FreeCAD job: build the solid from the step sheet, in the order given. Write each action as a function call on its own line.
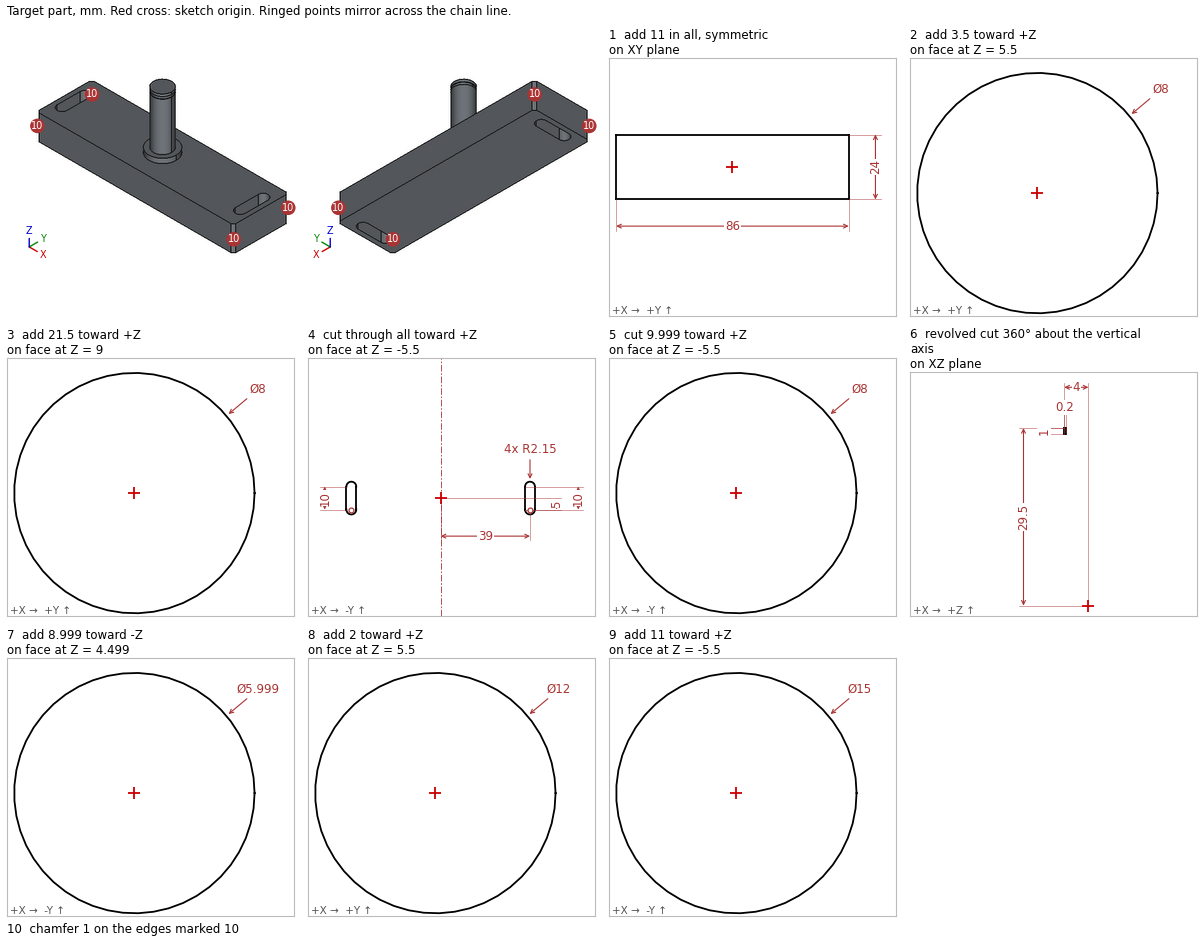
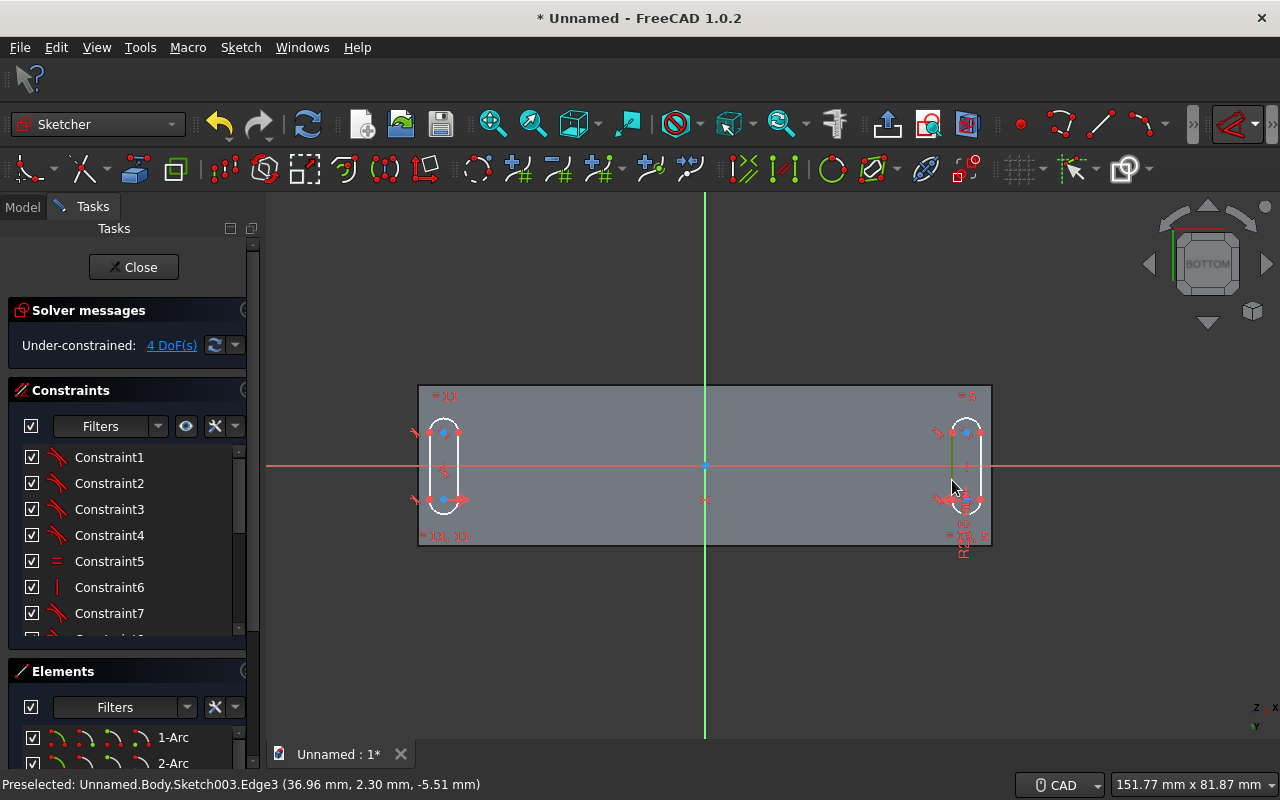
click(1258, 124)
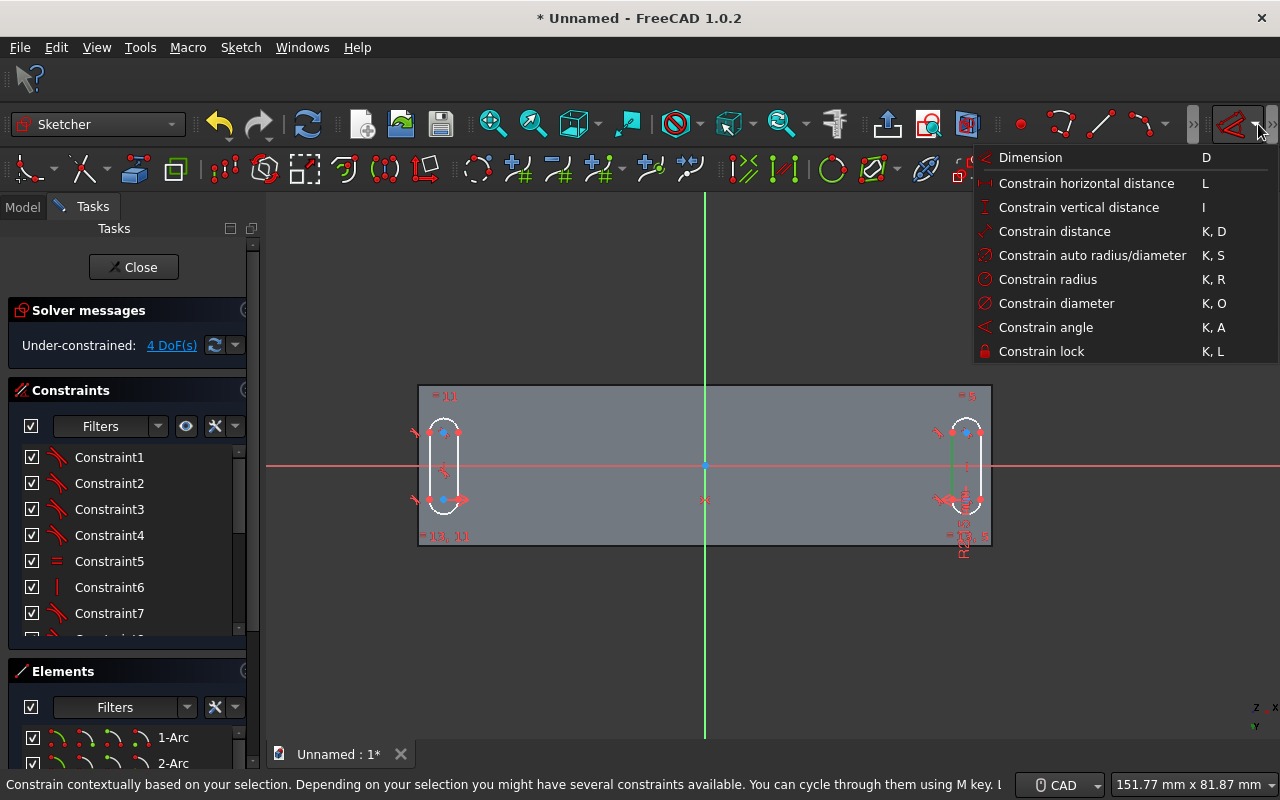
click(1126, 207)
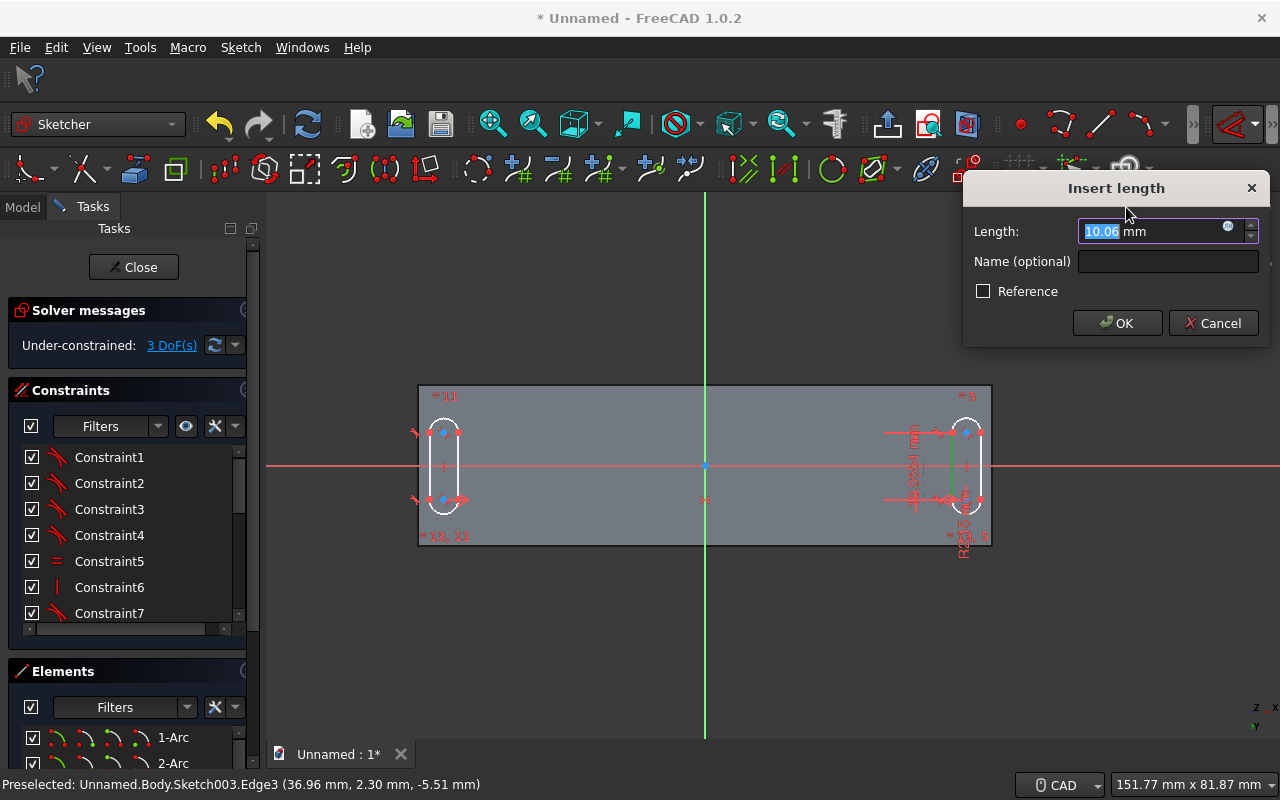
text(10)
key(Return)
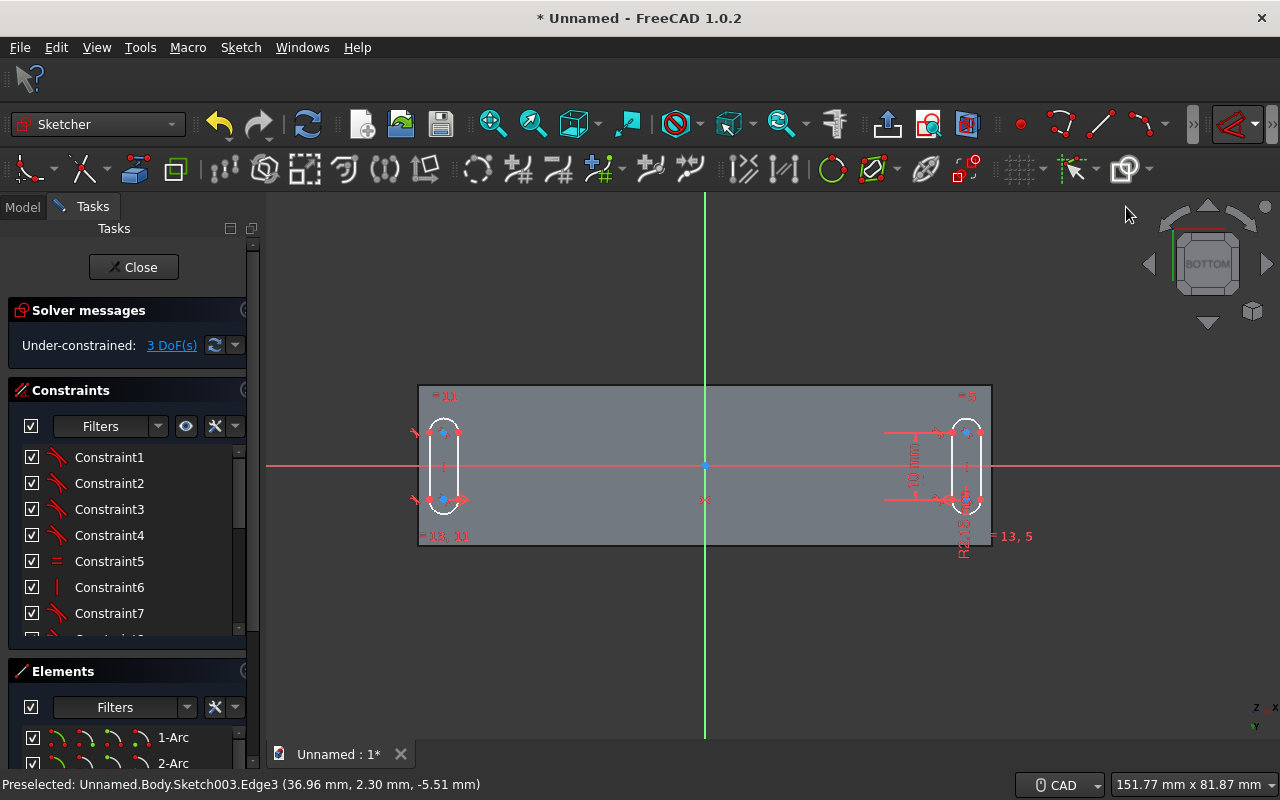
click(430, 480)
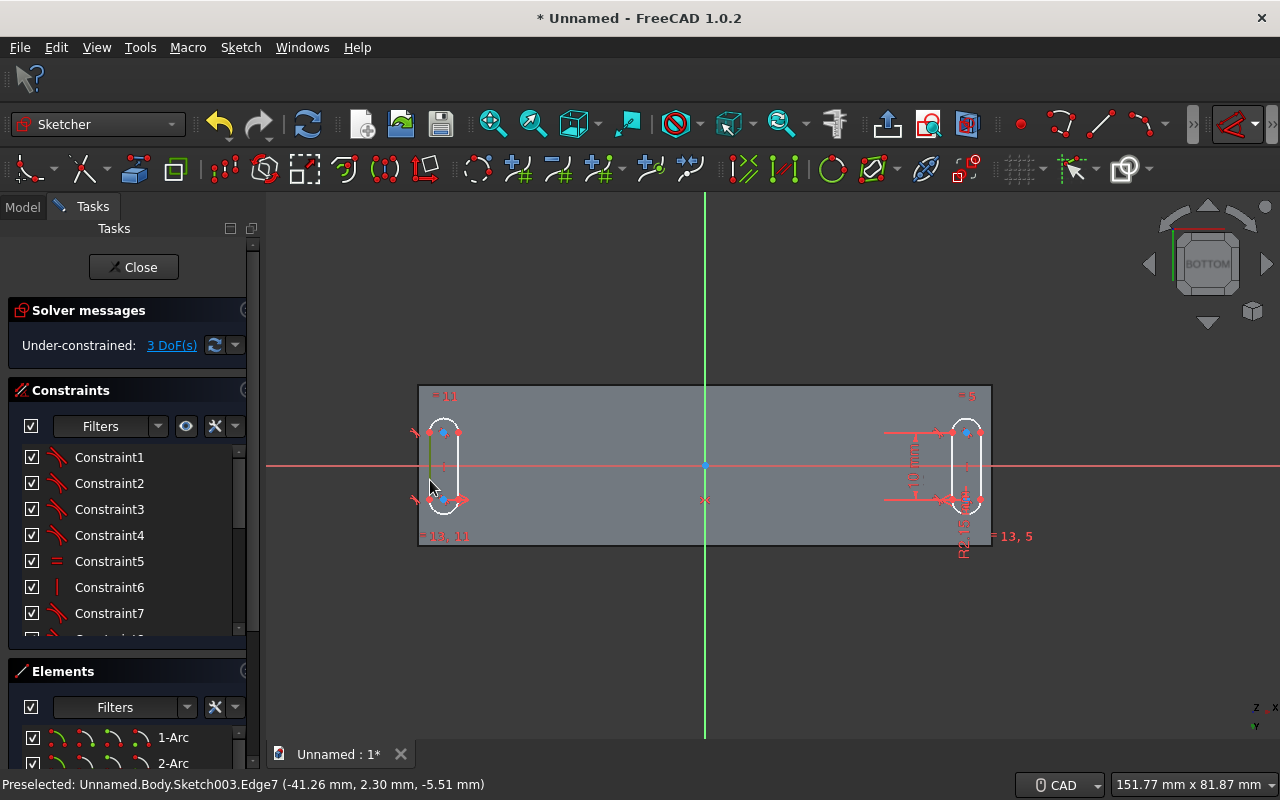
key(i)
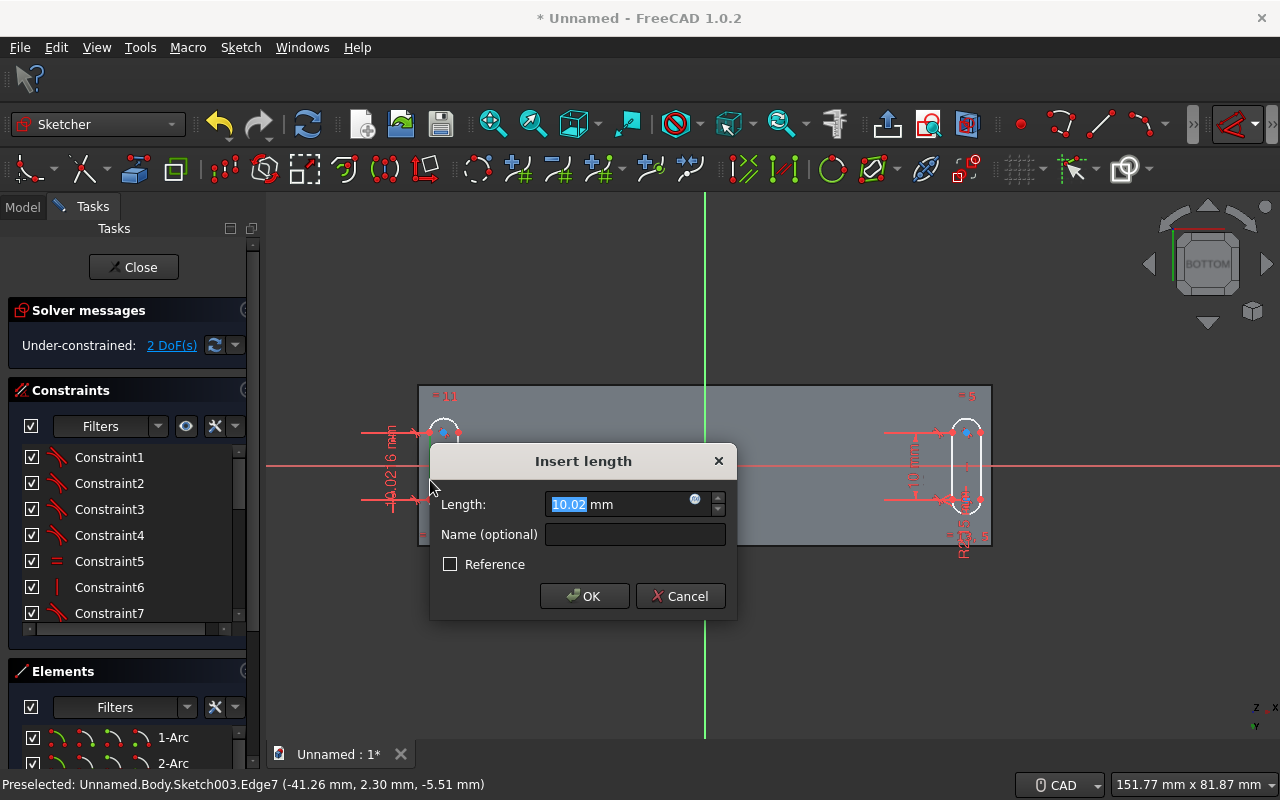
text(10)
key(Return)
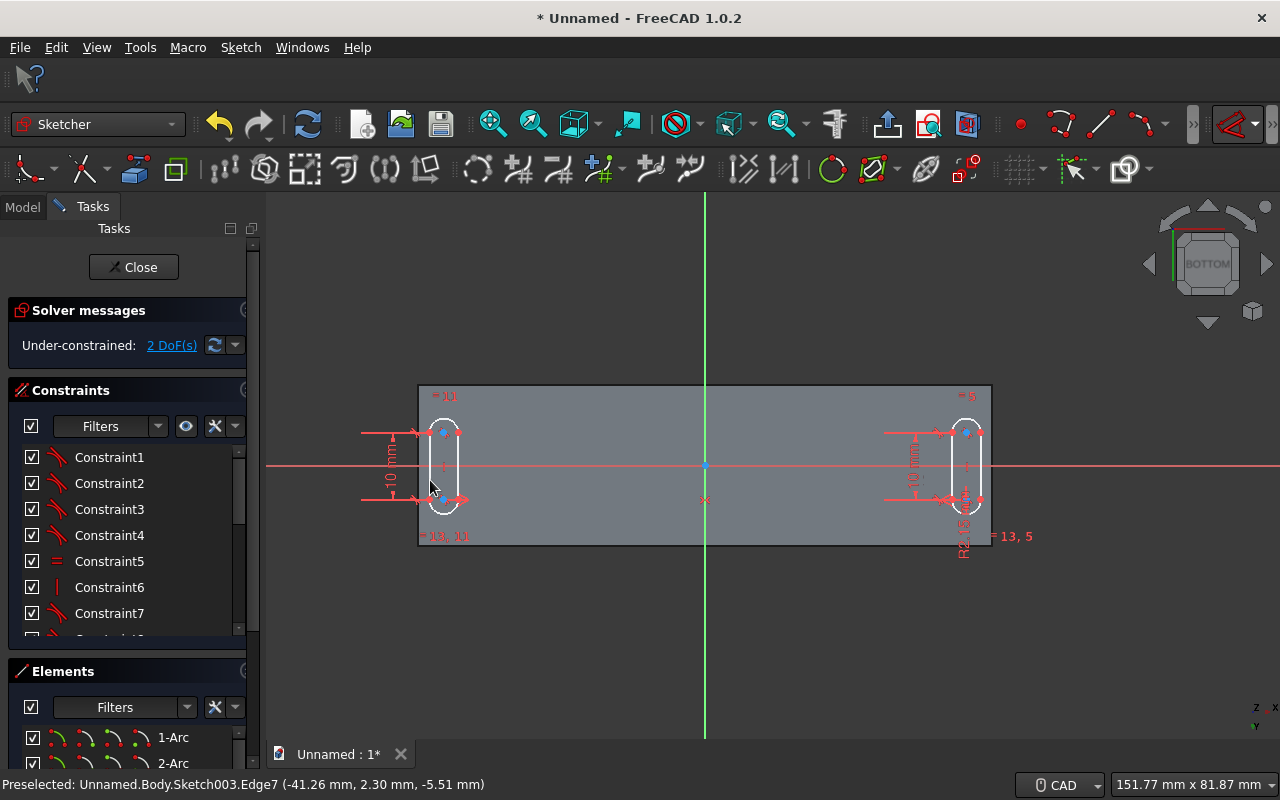
click(952, 500)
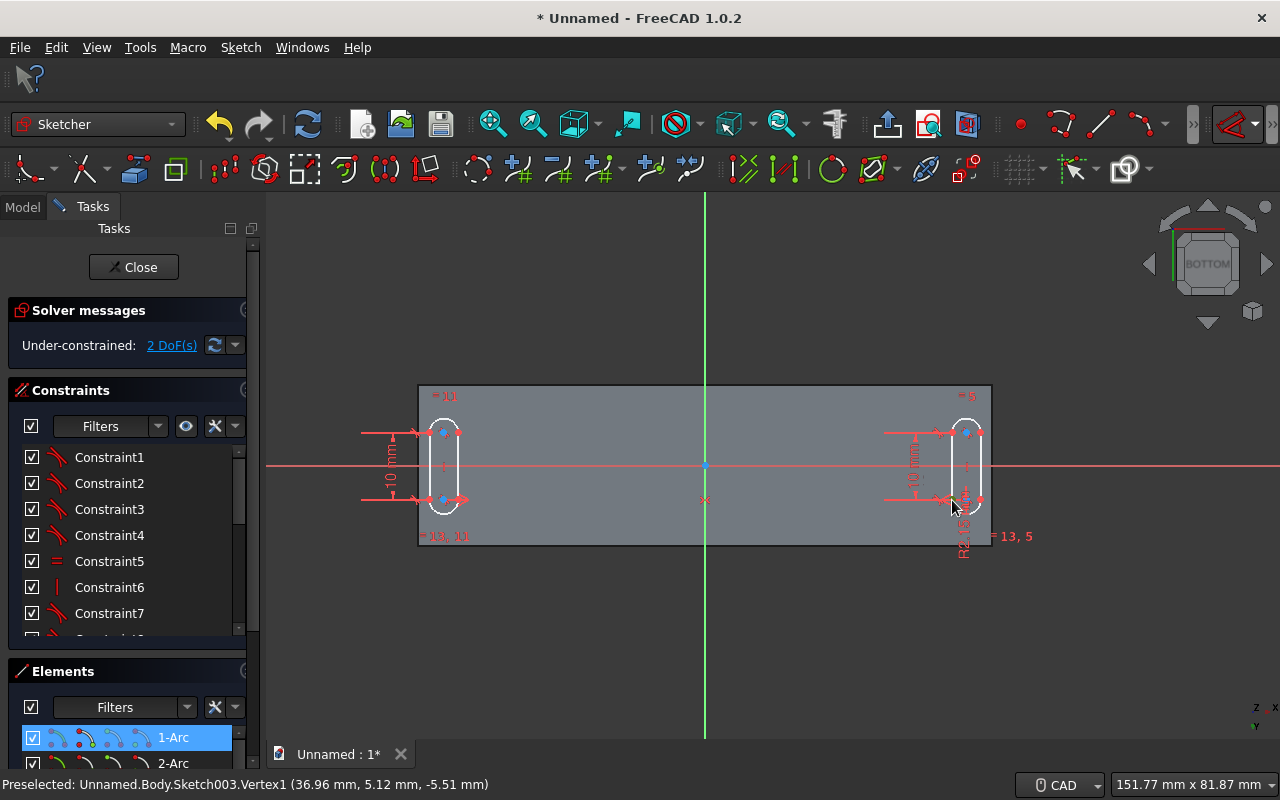
click(1258, 124)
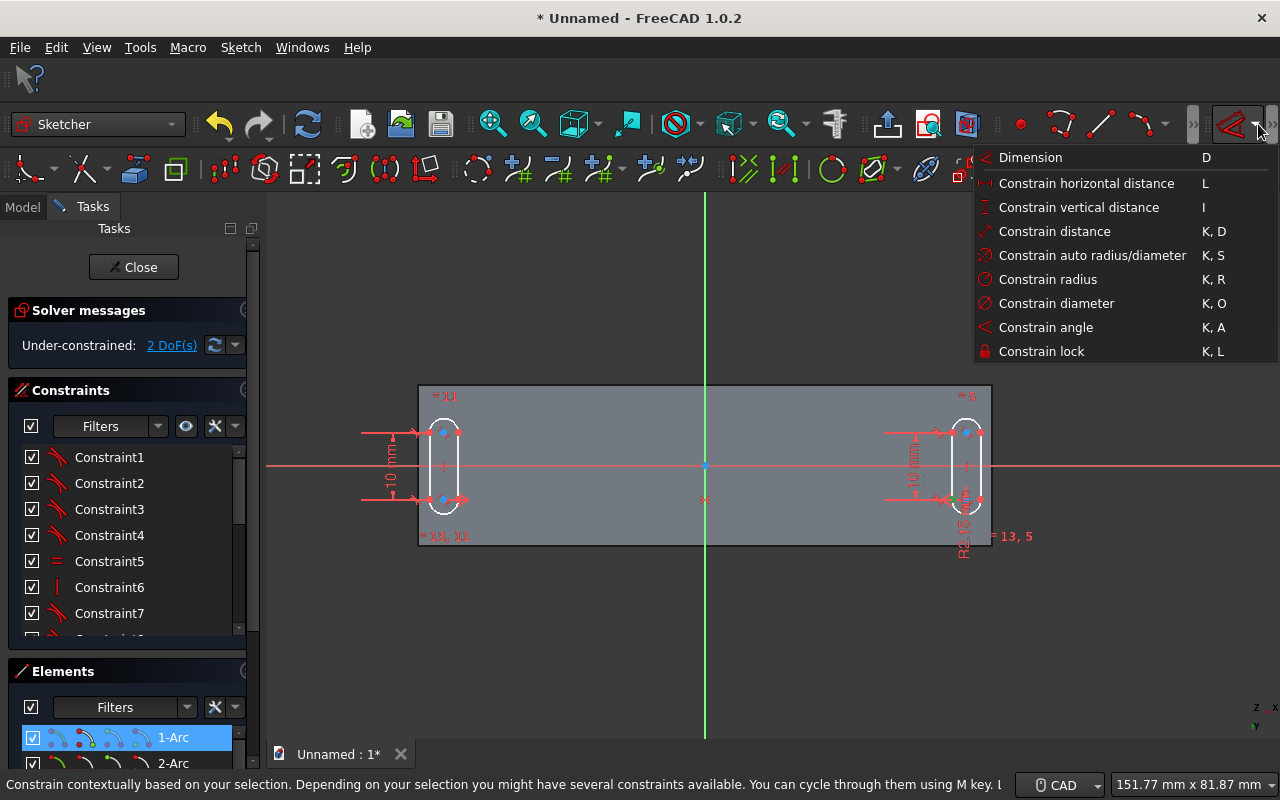
click(1126, 207)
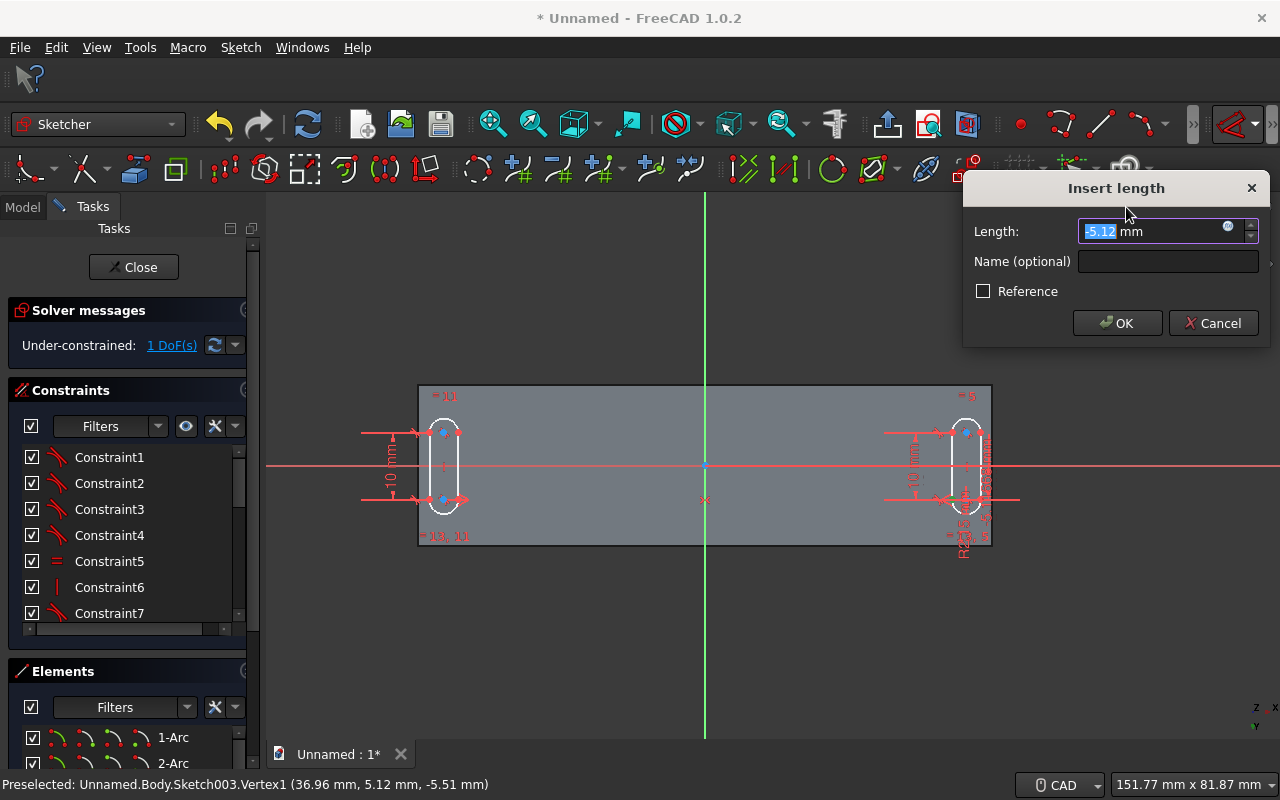
text(-5)
key(Return)